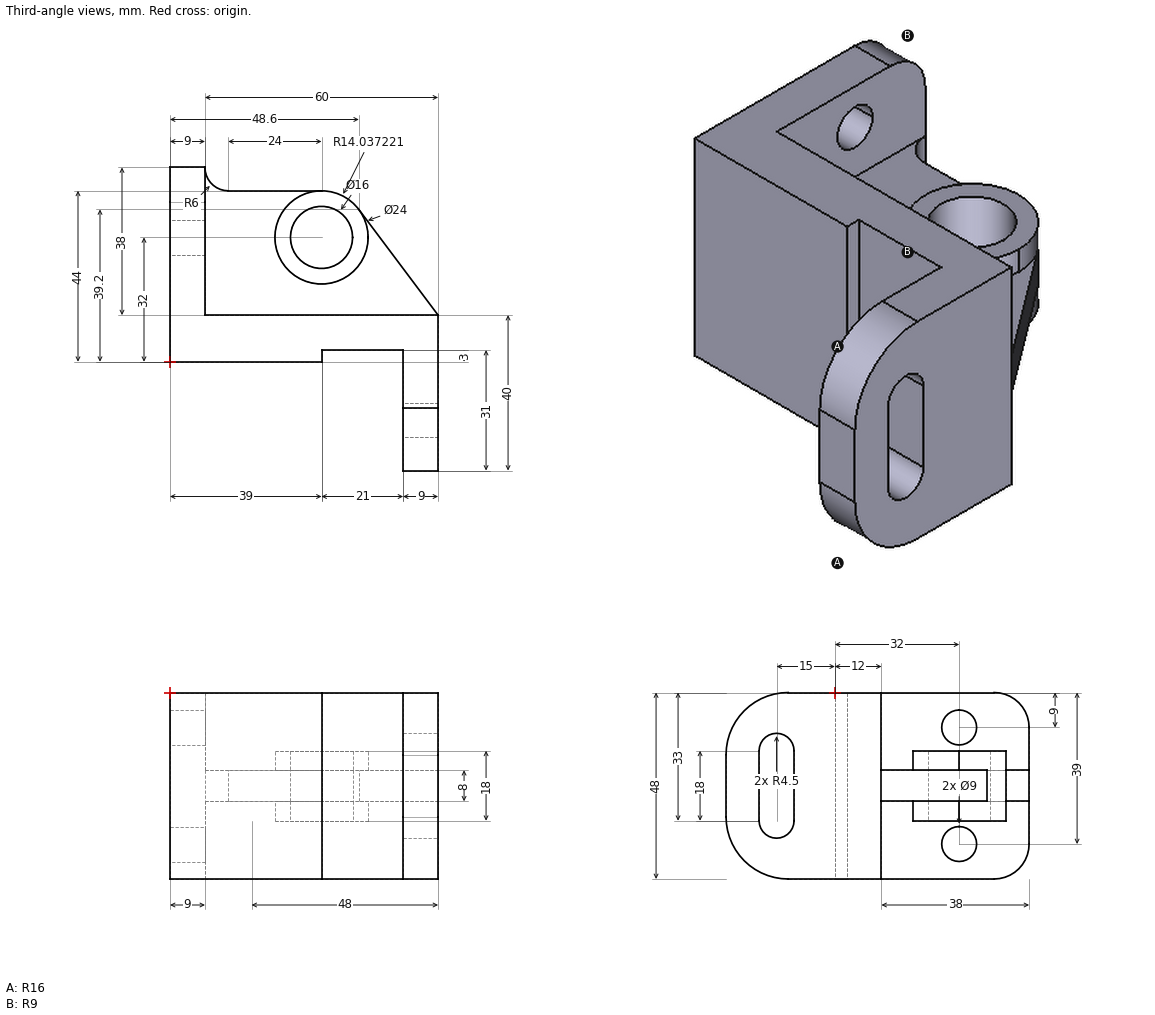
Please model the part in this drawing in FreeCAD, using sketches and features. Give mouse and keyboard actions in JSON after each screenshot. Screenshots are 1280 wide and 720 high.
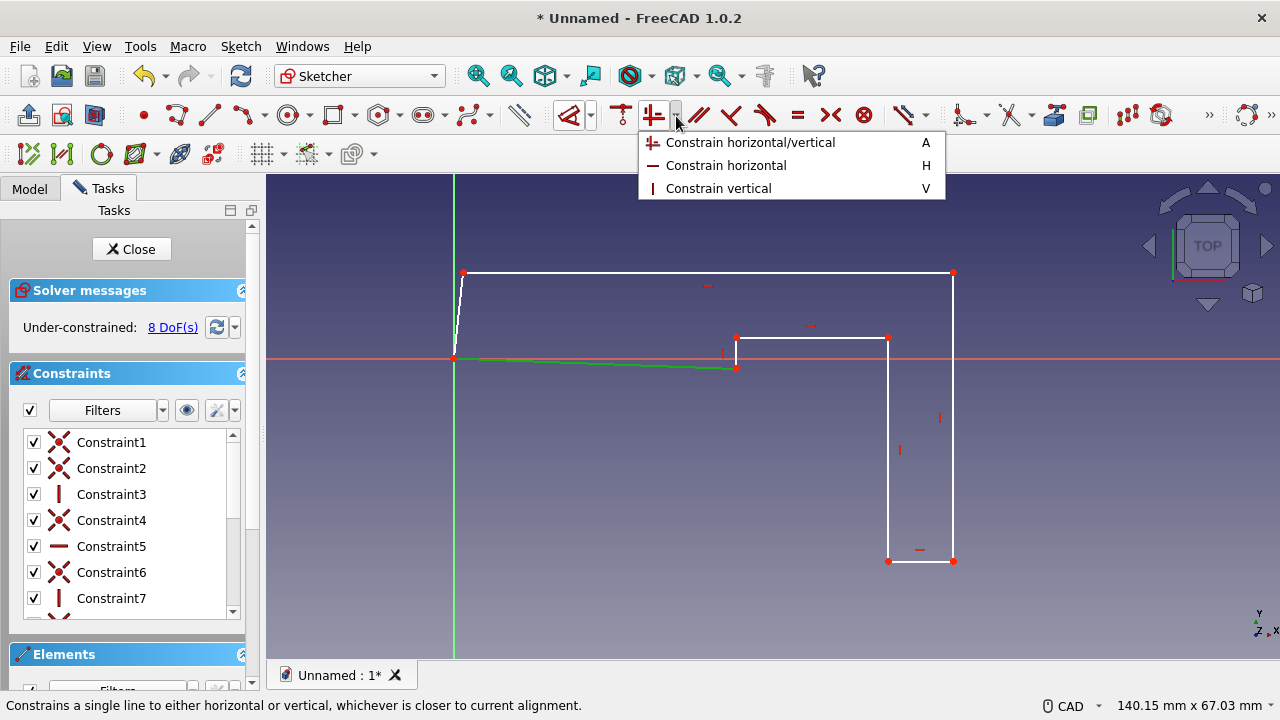
{"action": "left_click", "coordinate": [792, 166]}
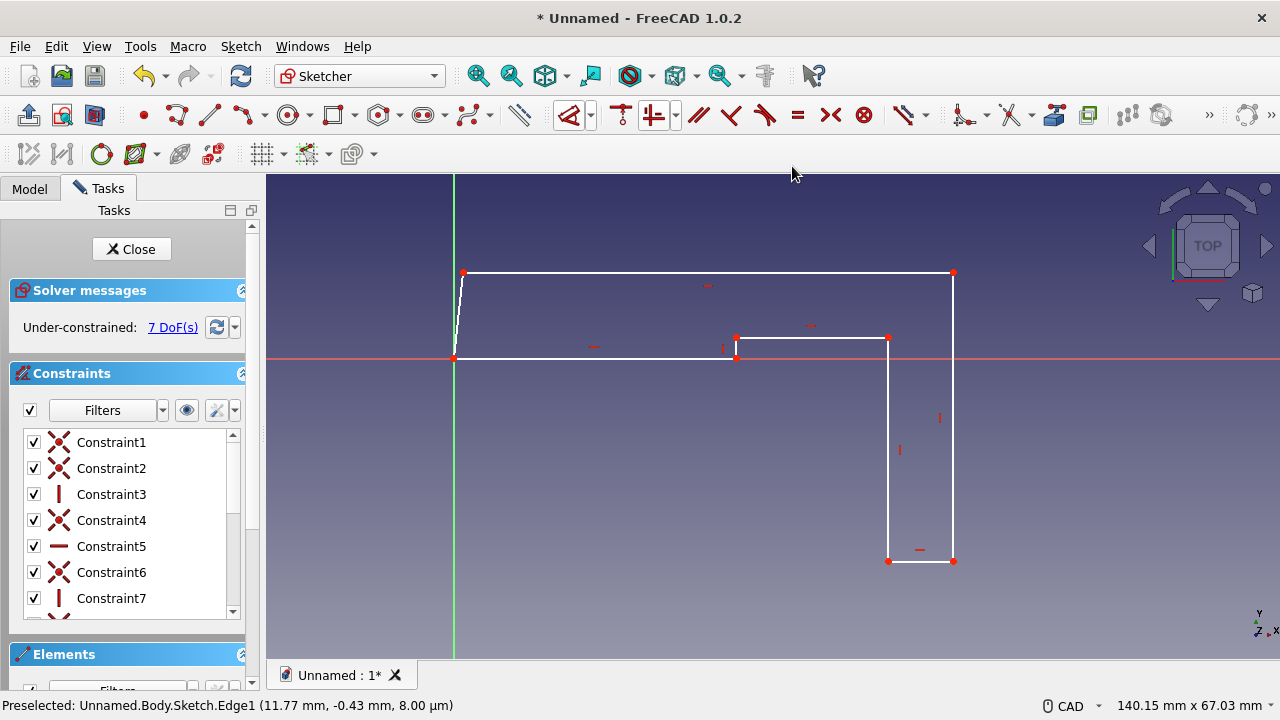
{"action": "left_click", "coordinate": [457, 333]}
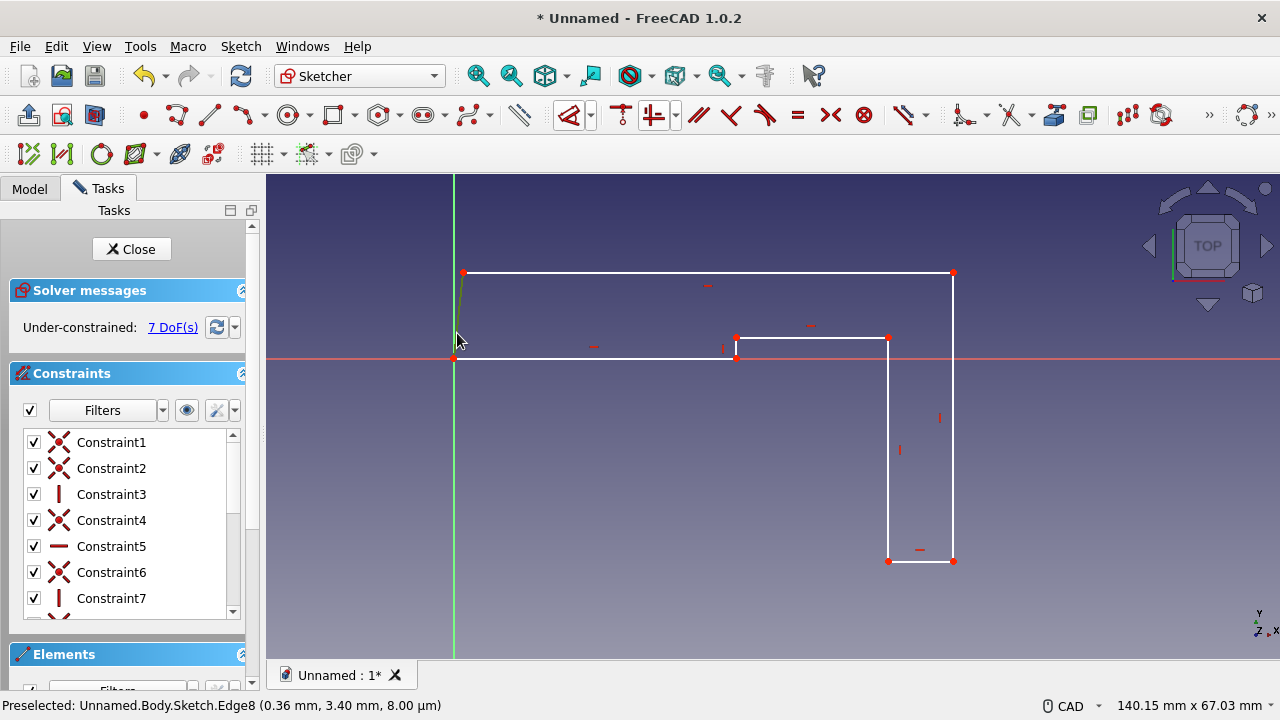
{"action": "key", "text": "v"}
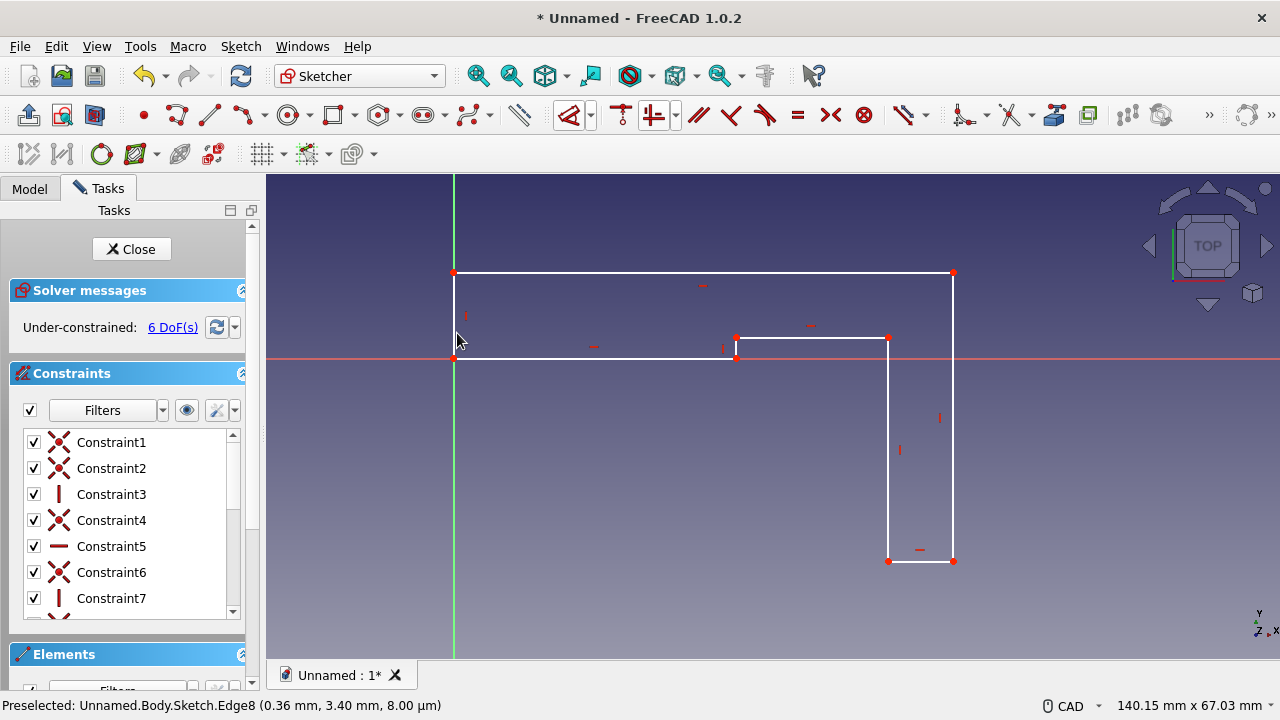
{"action": "key", "text": "d"}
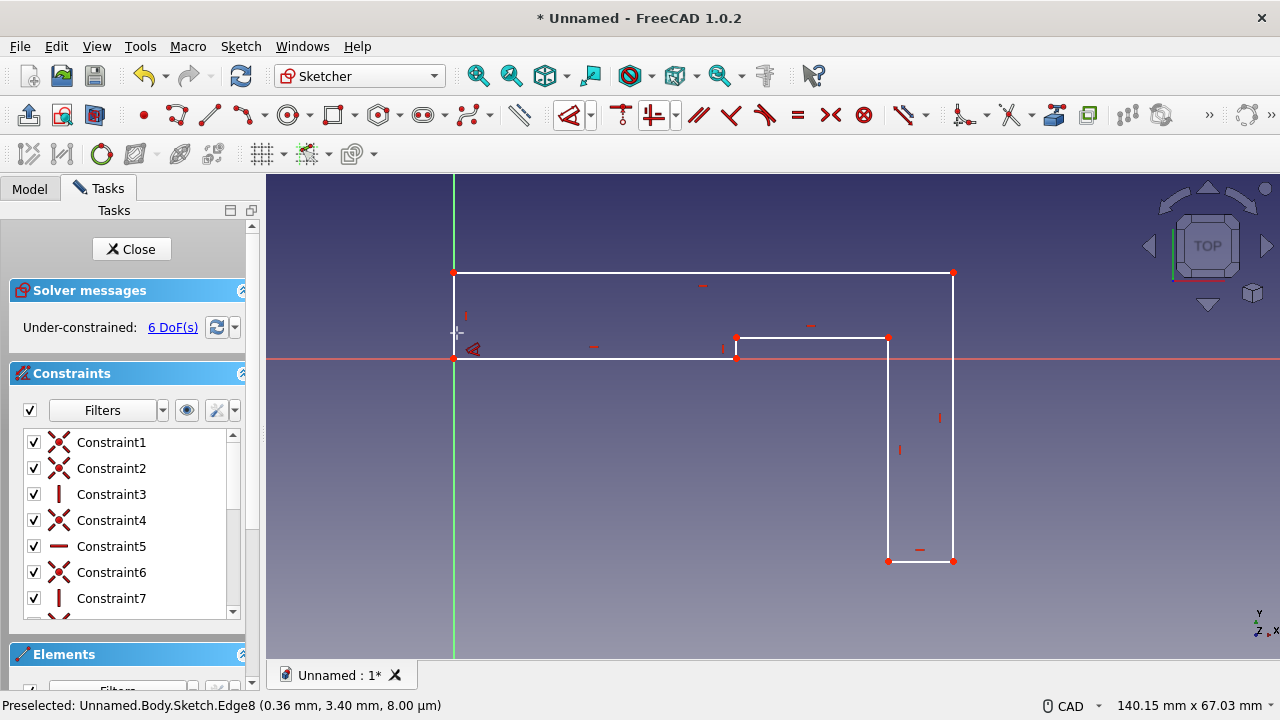
{"action": "scroll", "coordinate": [736, 348], "scroll_direction": "up", "scroll_amount": 4}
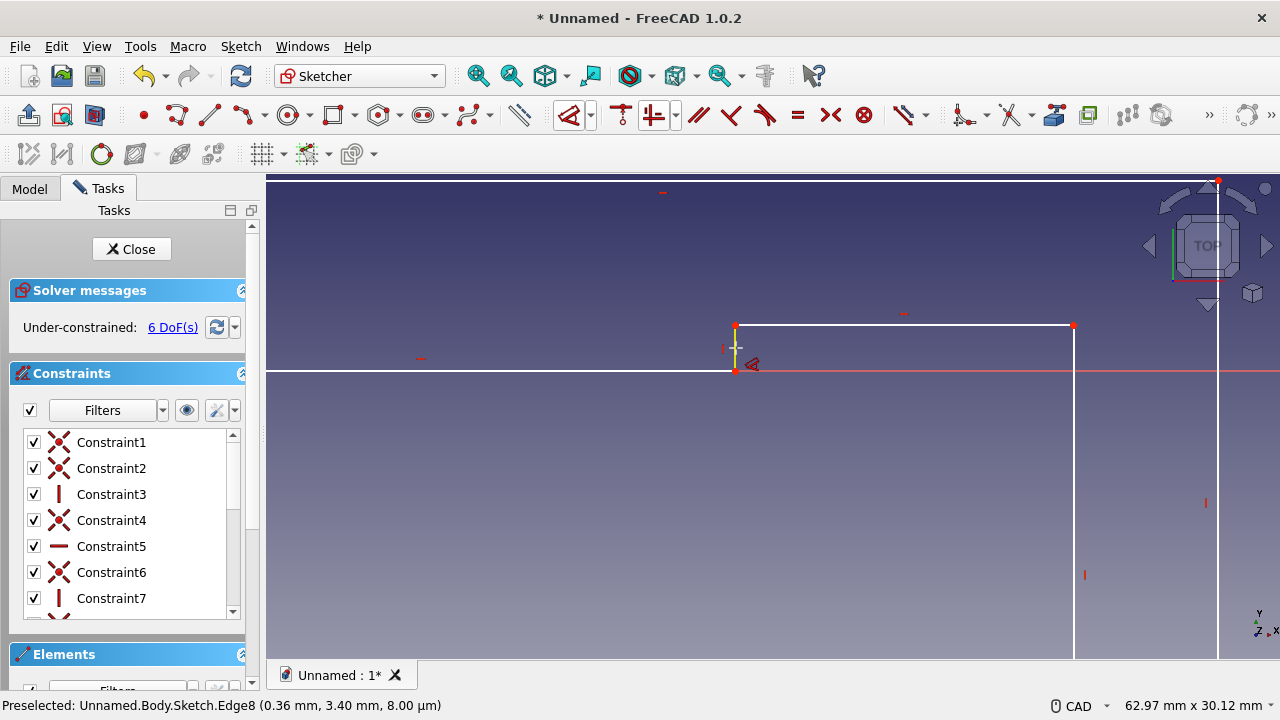
{"action": "left_click", "coordinate": [735, 348]}
{"action": "left_click", "coordinate": [769, 348]}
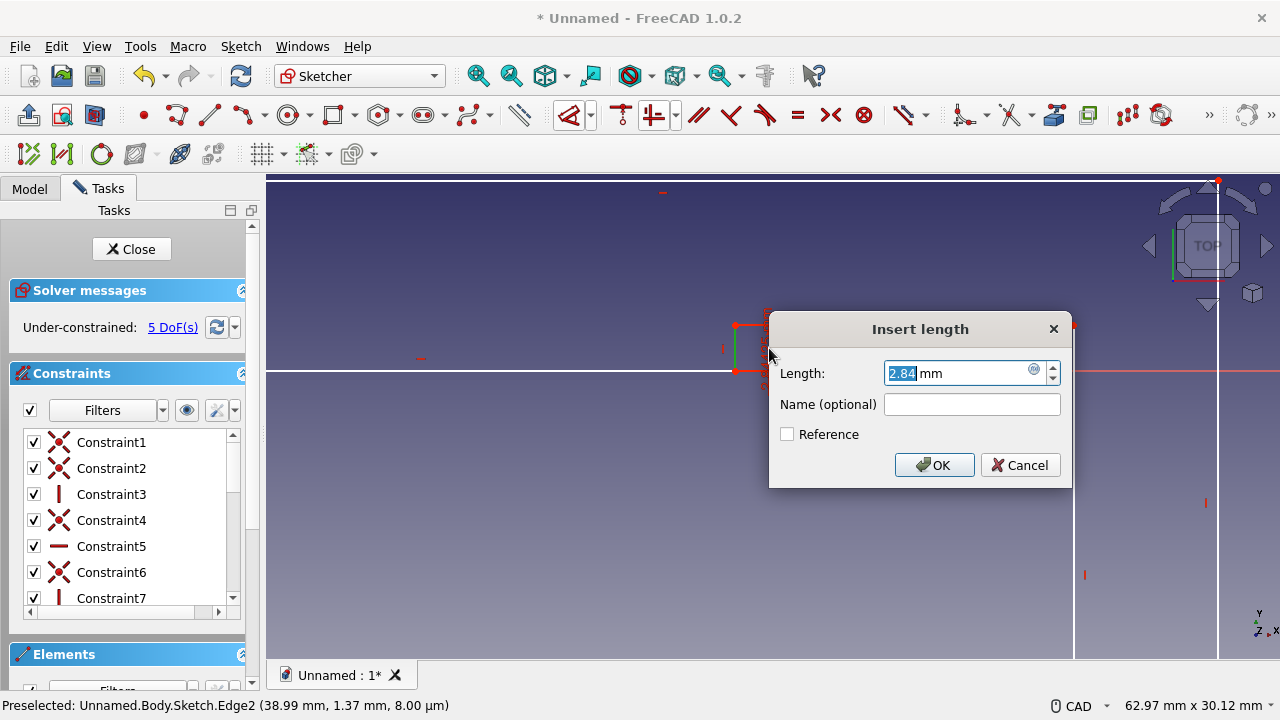
{"action": "type", "text": "3"}
{"action": "key", "text": "Return"}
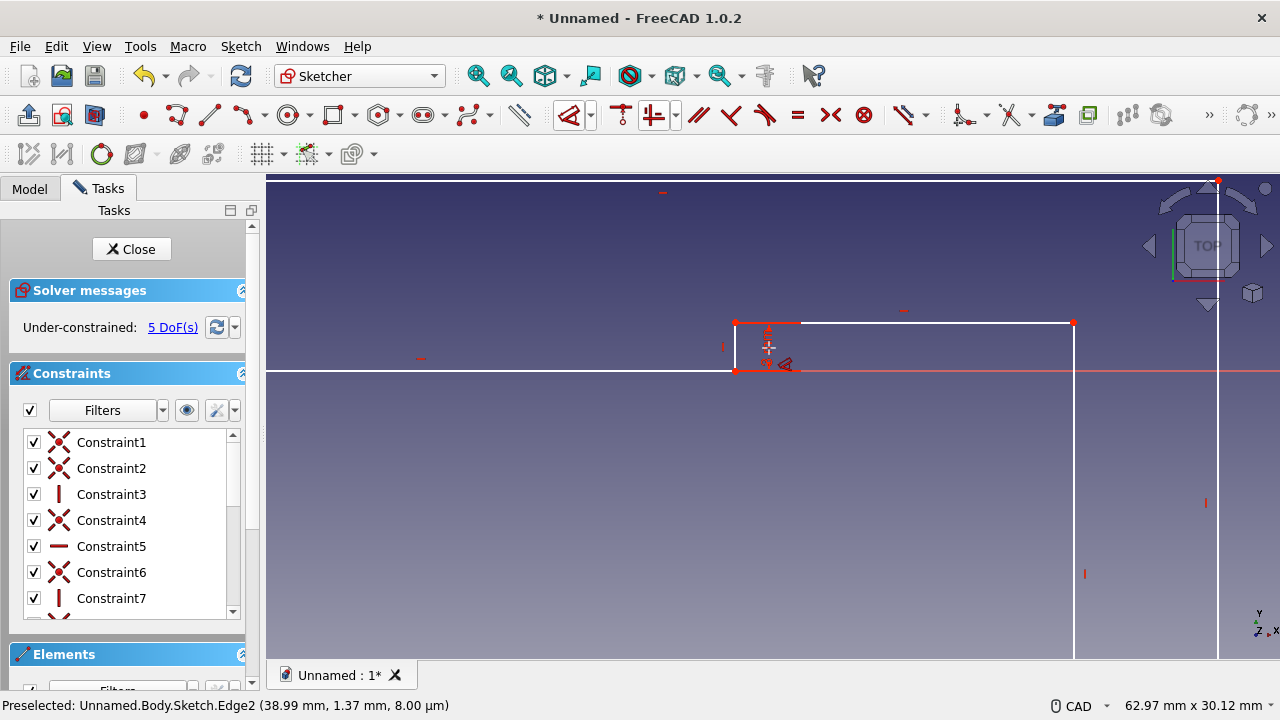
{"action": "scroll", "coordinate": [738, 348], "scroll_direction": "down", "scroll_amount": 4}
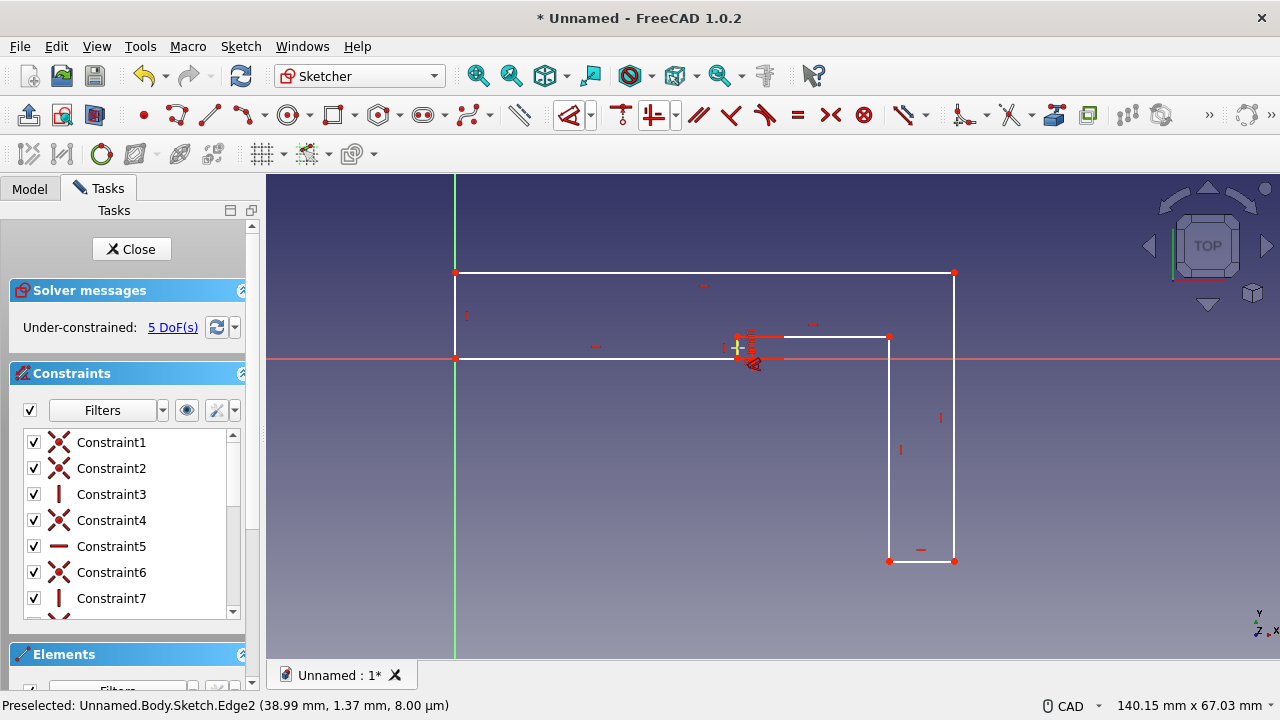
{"action": "left_click", "coordinate": [909, 562]}
{"action": "left_click", "coordinate": [922, 596]}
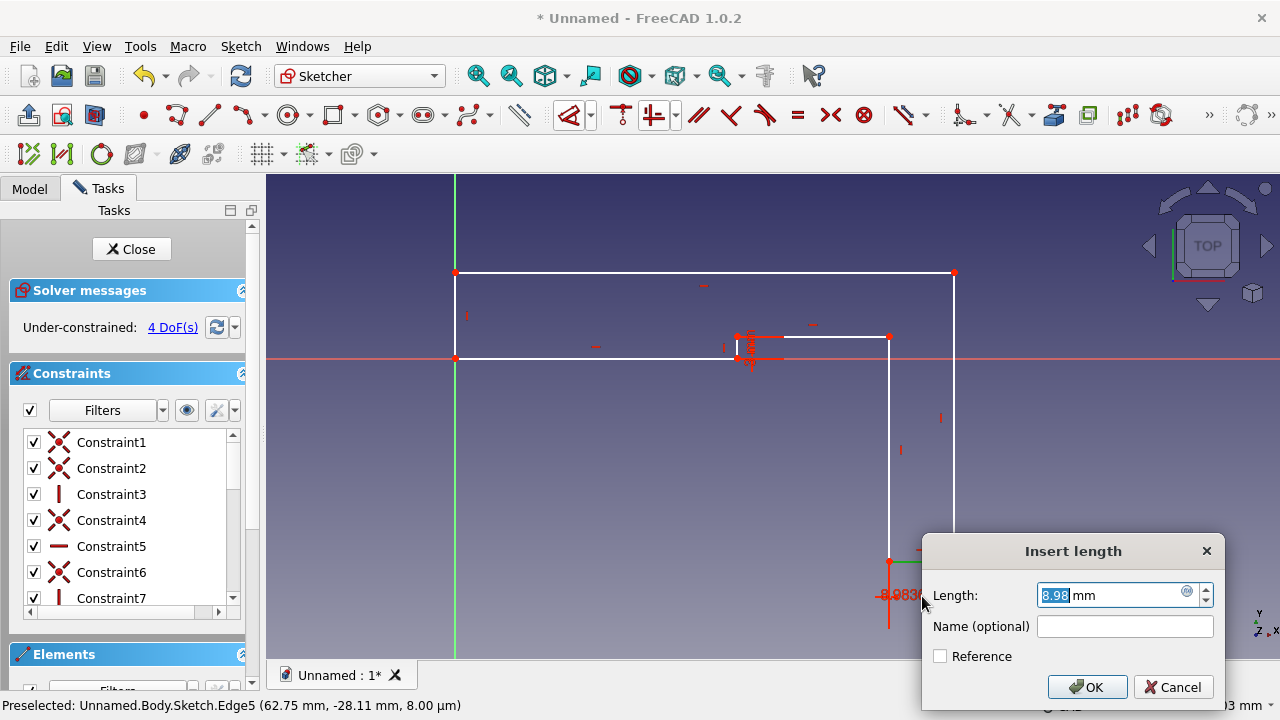
{"action": "type", "text": "9"}
{"action": "key", "text": "Return"}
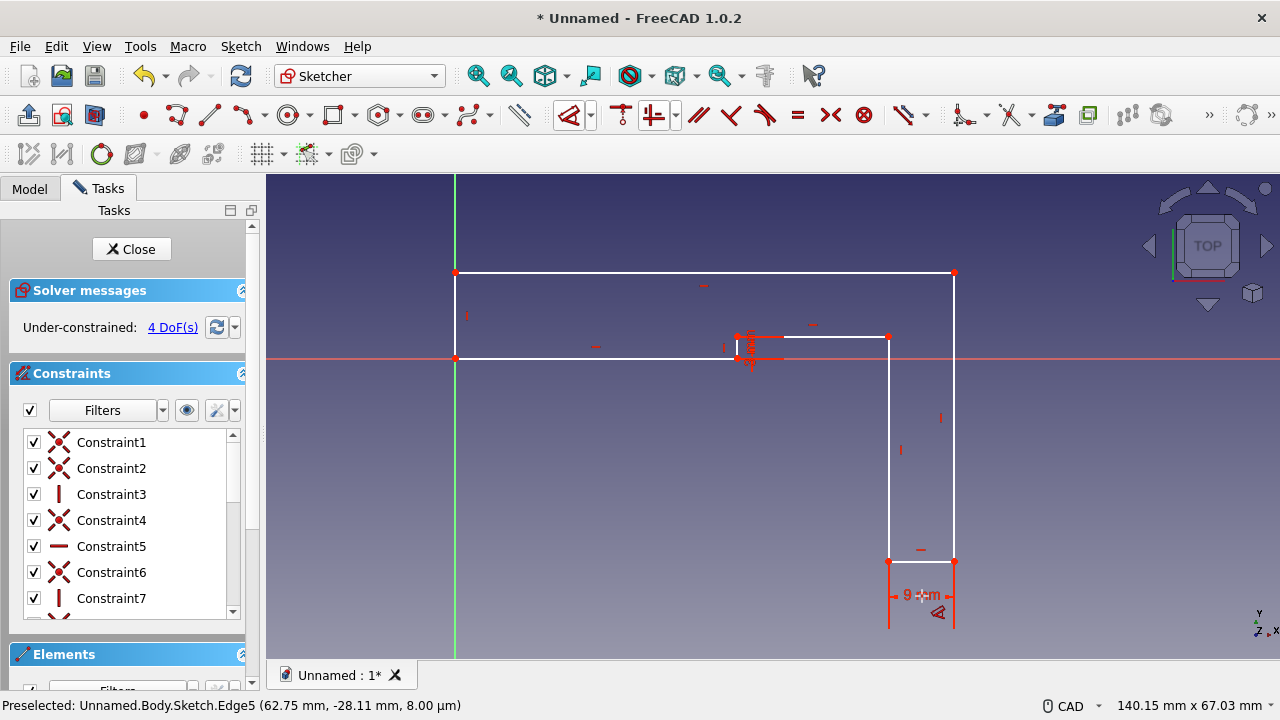
{"action": "left_click", "coordinate": [540, 359]}
{"action": "left_click", "coordinate": [596, 325]}